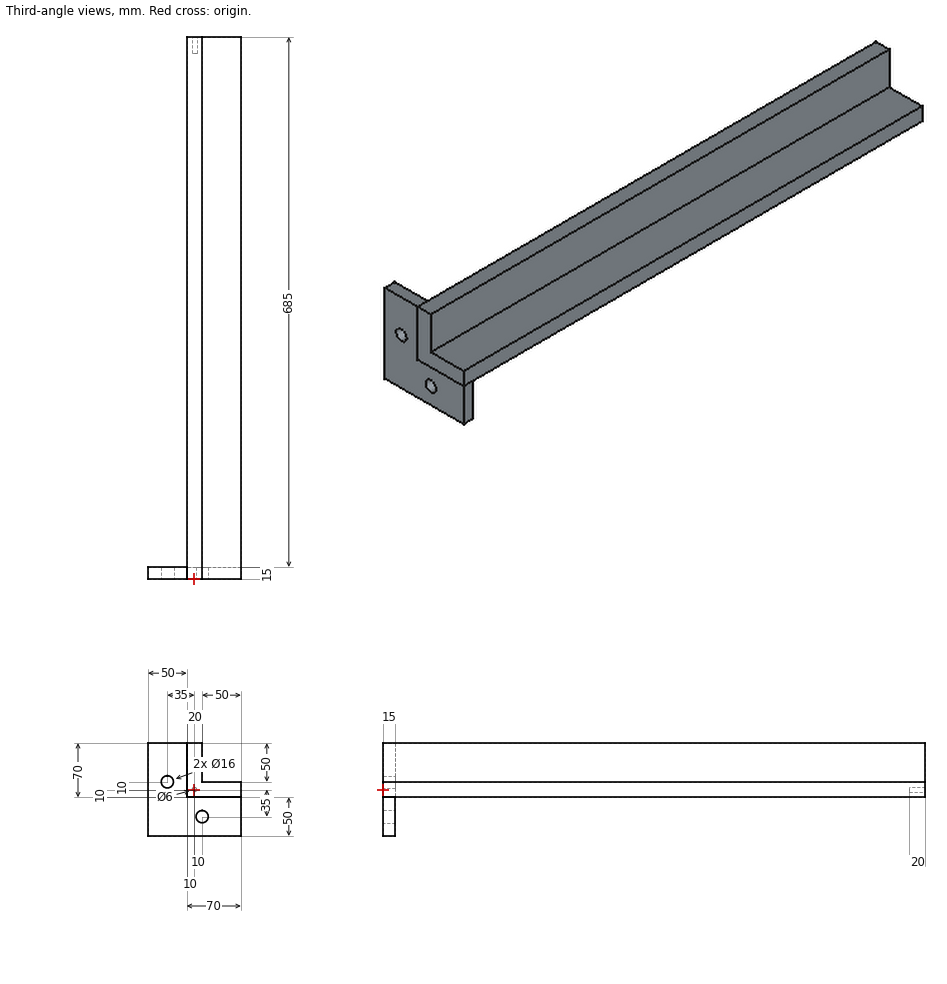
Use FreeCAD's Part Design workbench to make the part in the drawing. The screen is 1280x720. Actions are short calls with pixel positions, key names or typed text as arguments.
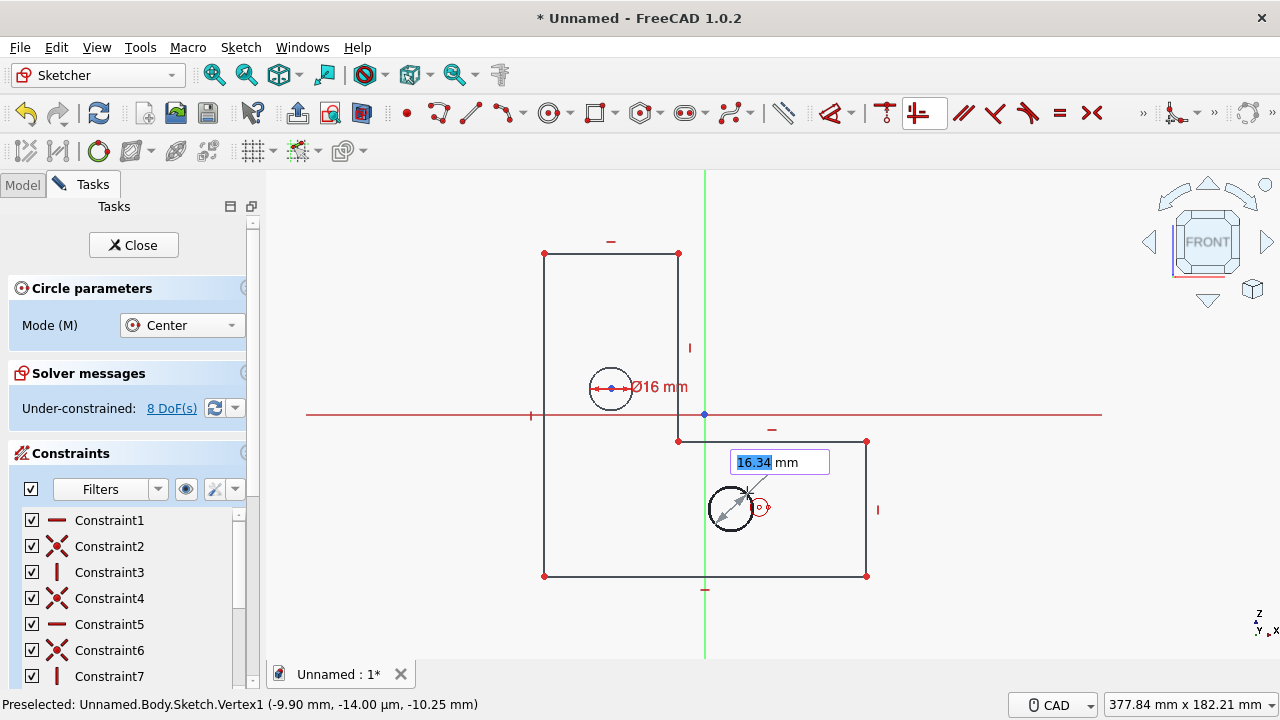
text(16)
key(Return)
key(Escape)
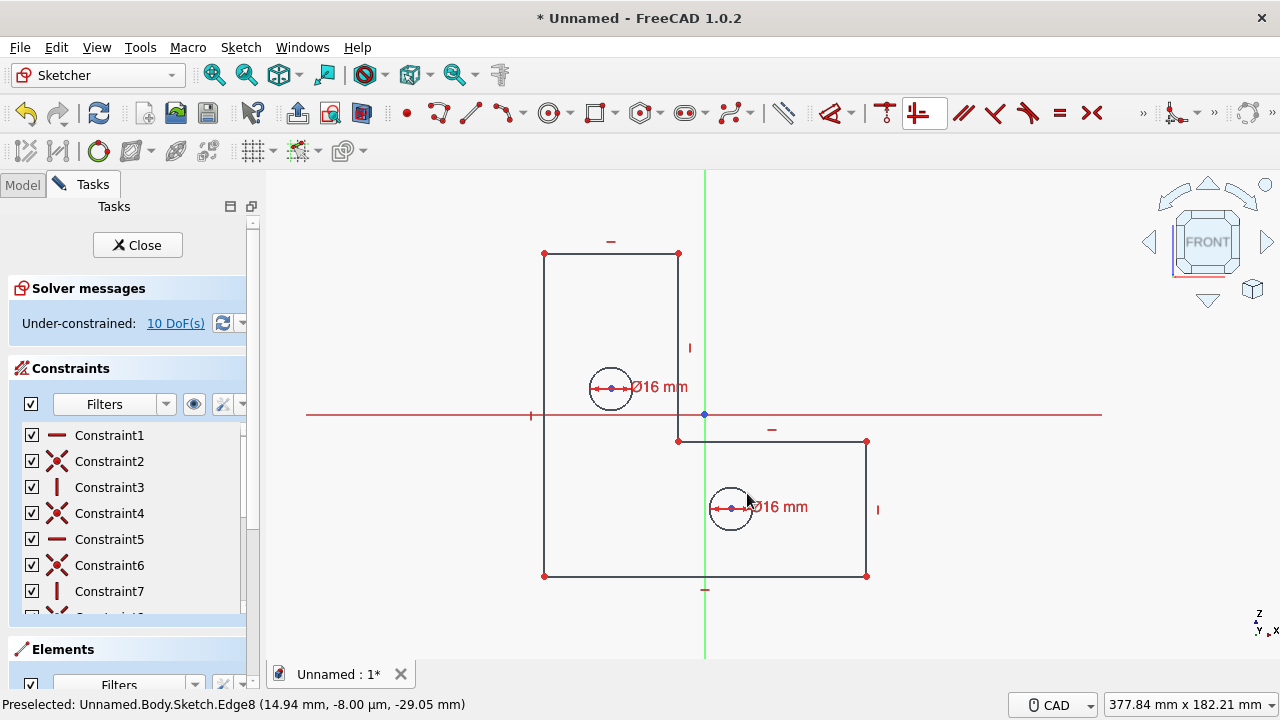
click(734, 442)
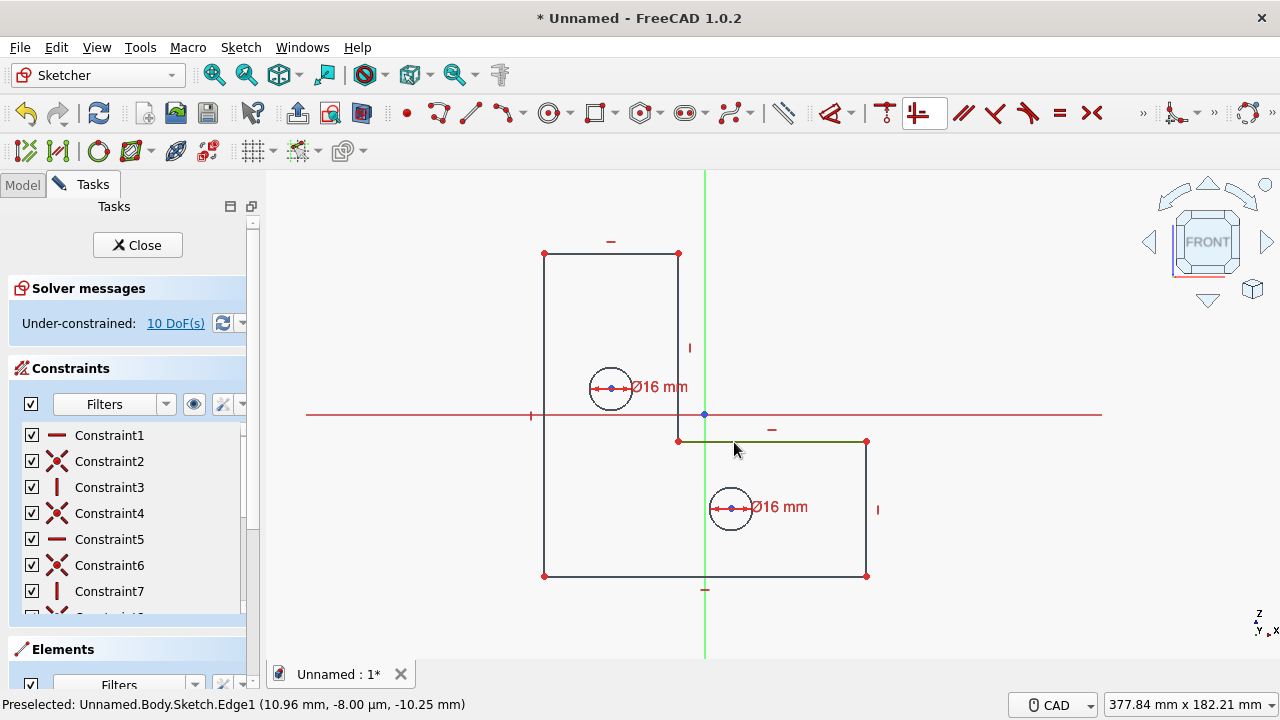
click(854, 114)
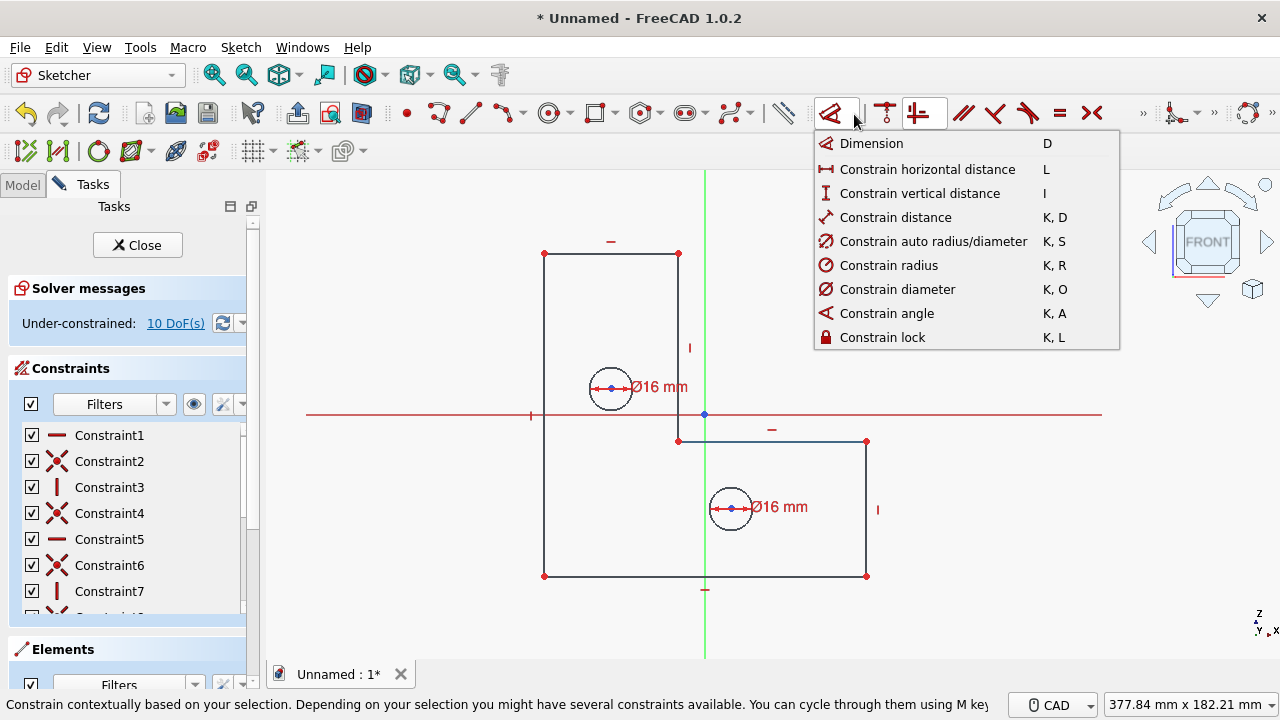
click(967, 169)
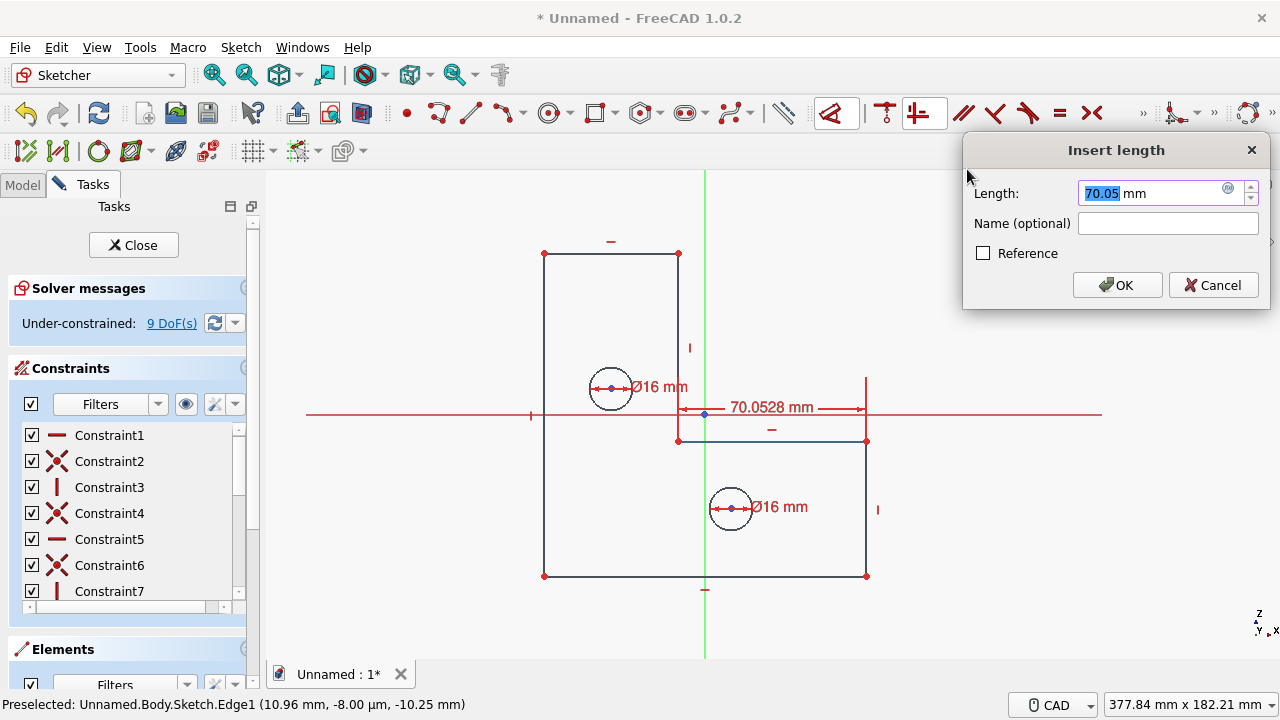
text(70)
key(Return)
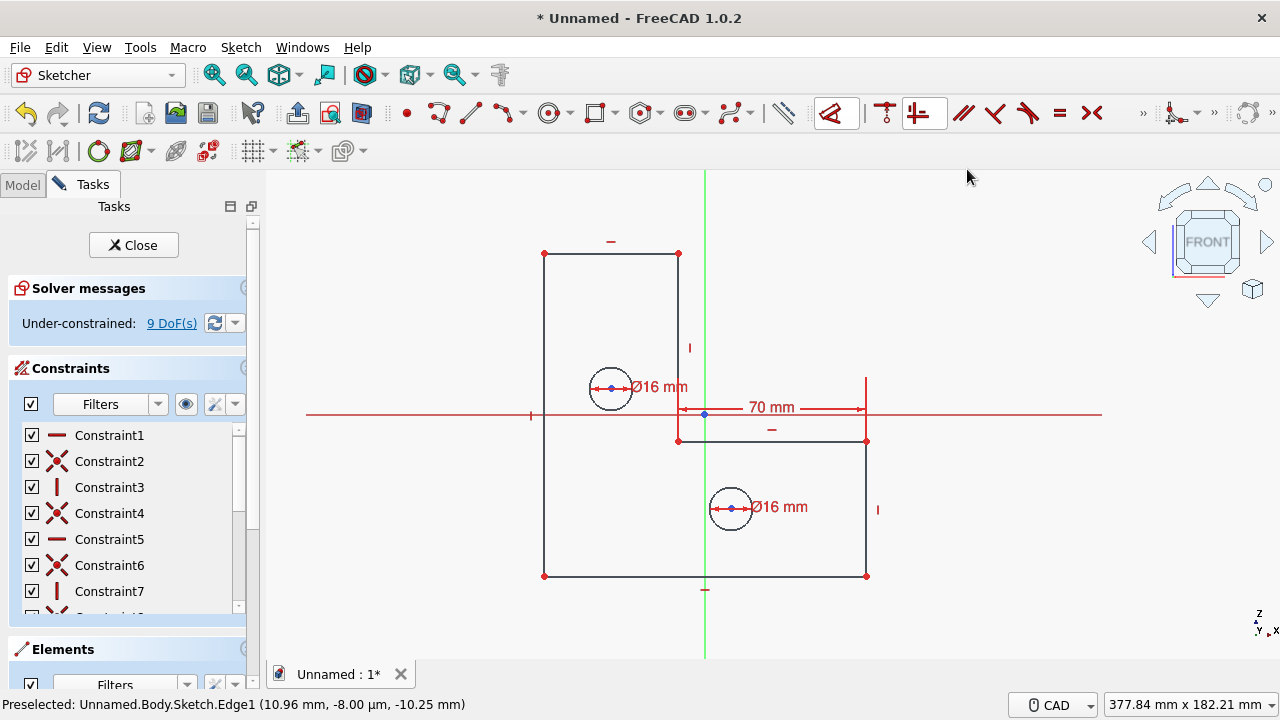
click(866, 483)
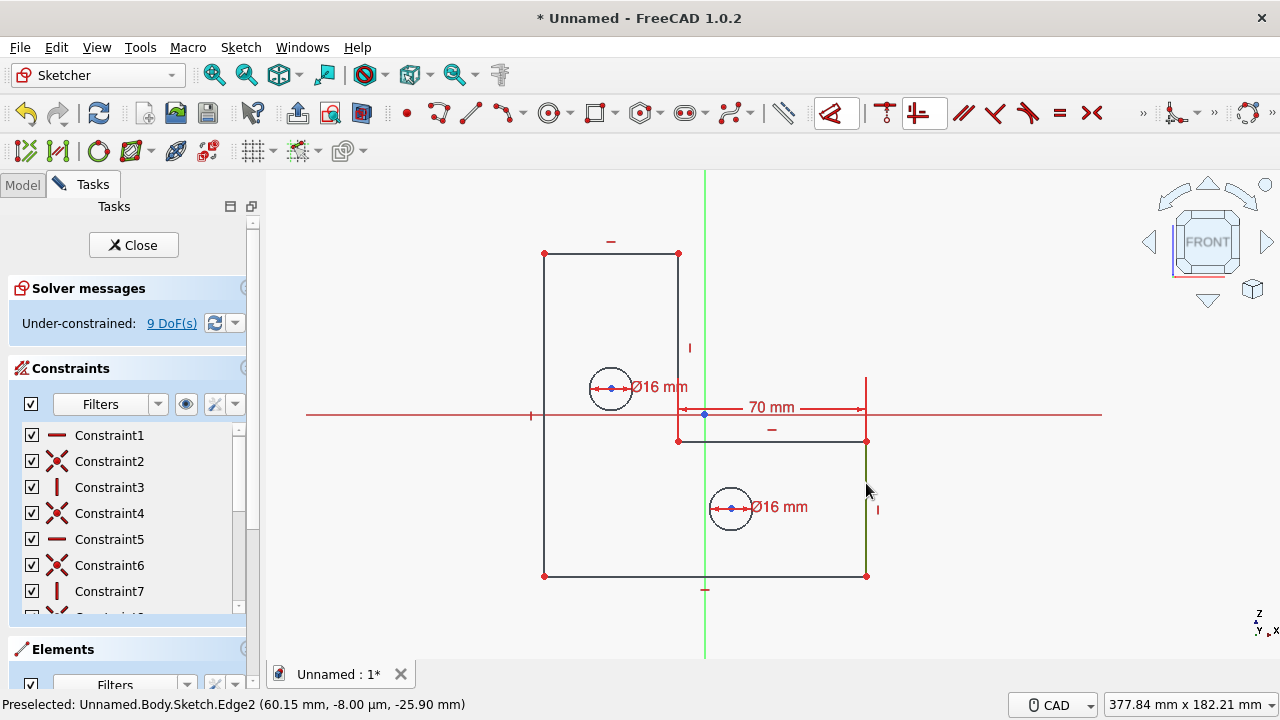
key(i)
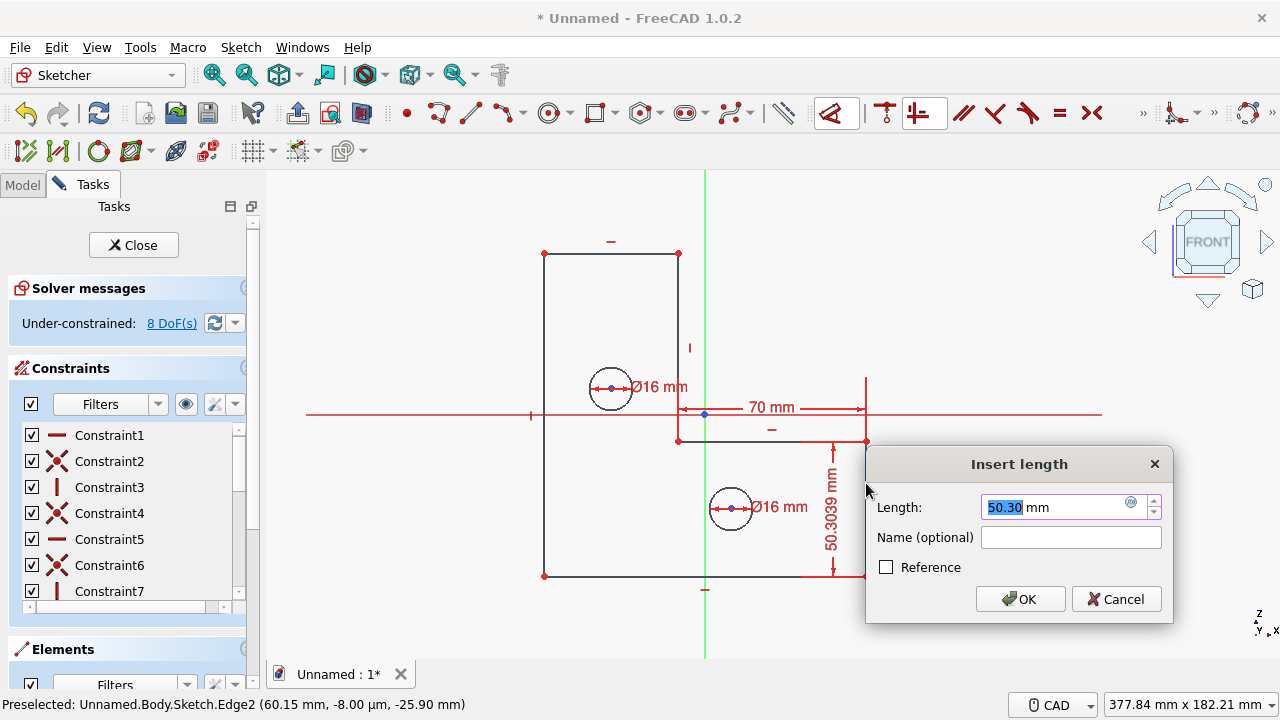
text(50)
key(Return)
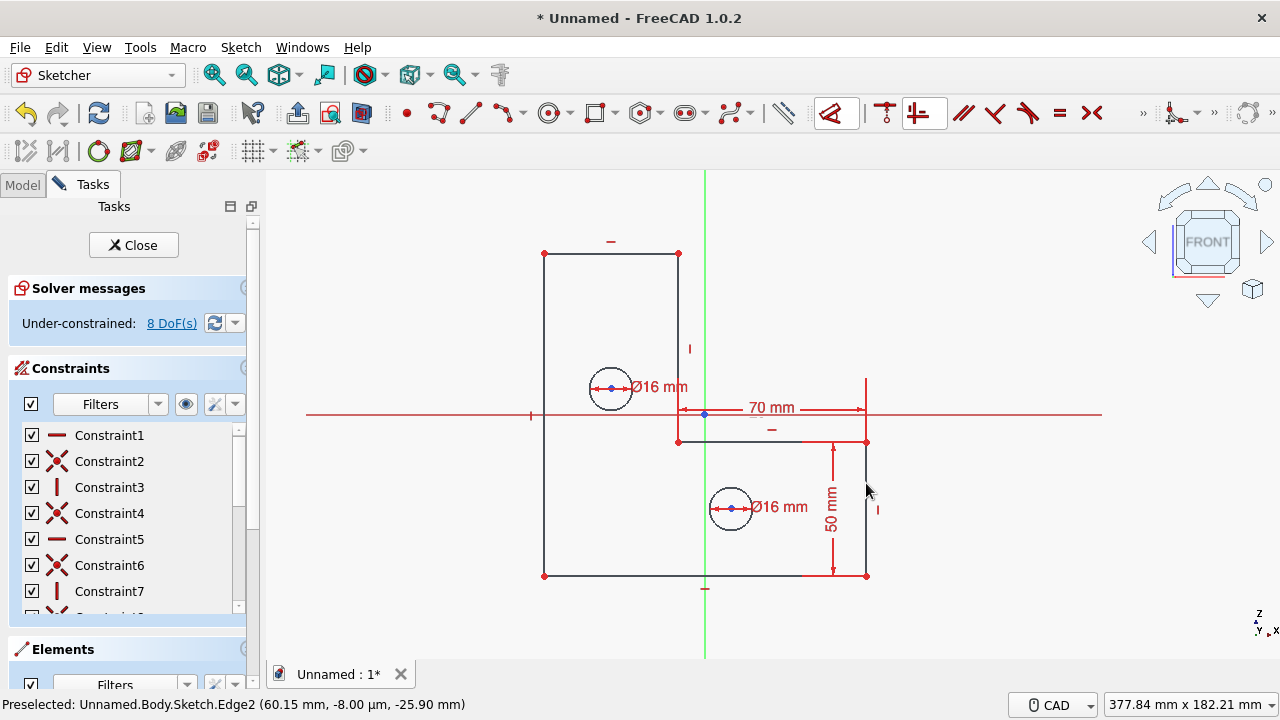
click(584, 254)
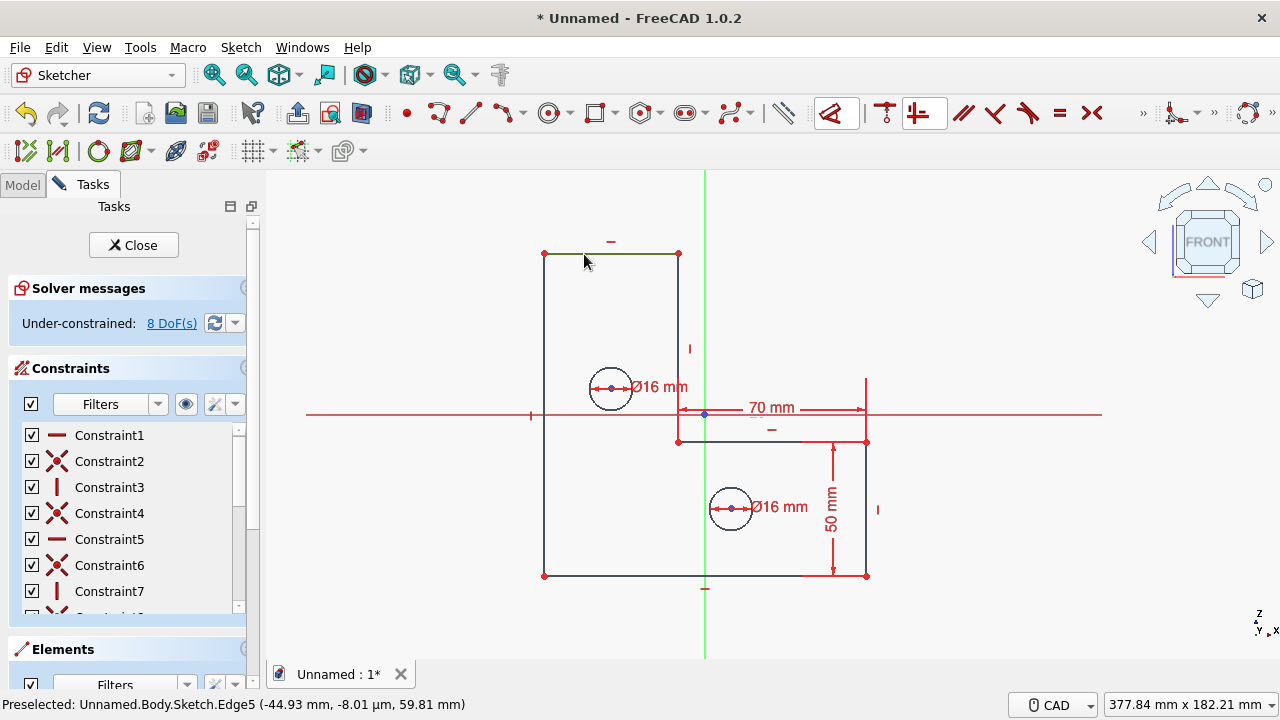
click(854, 114)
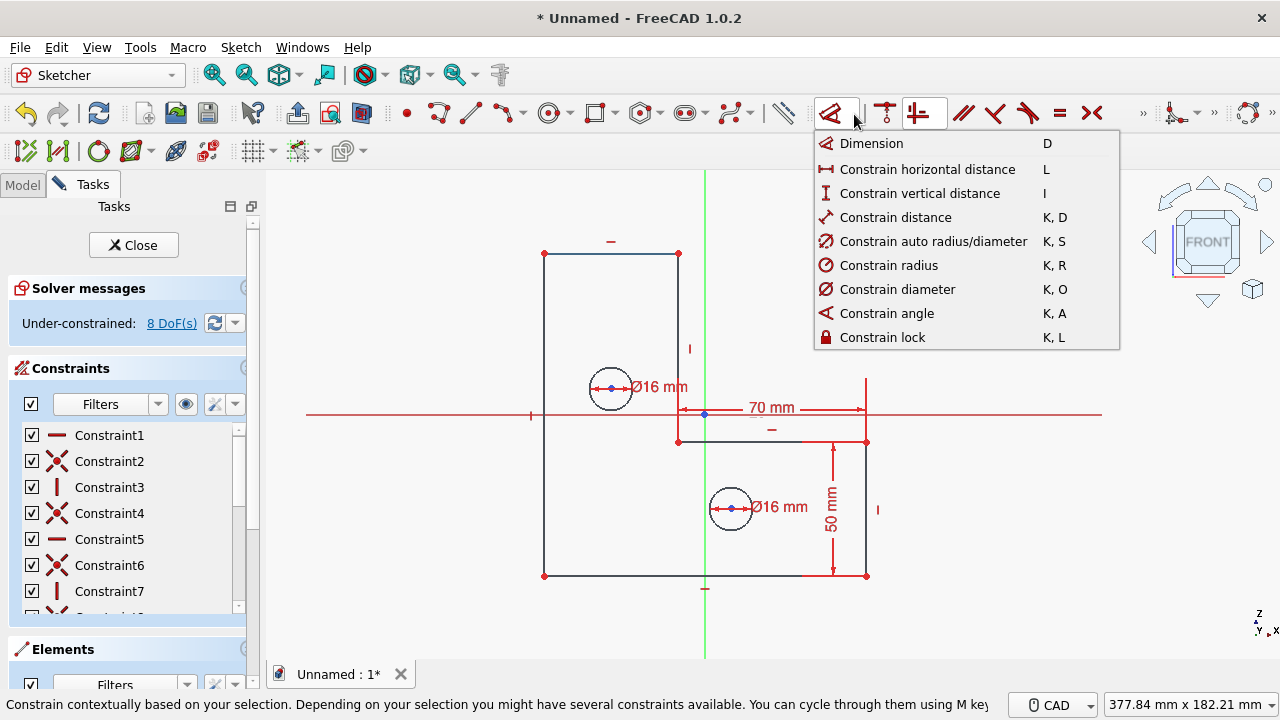
click(967, 169)